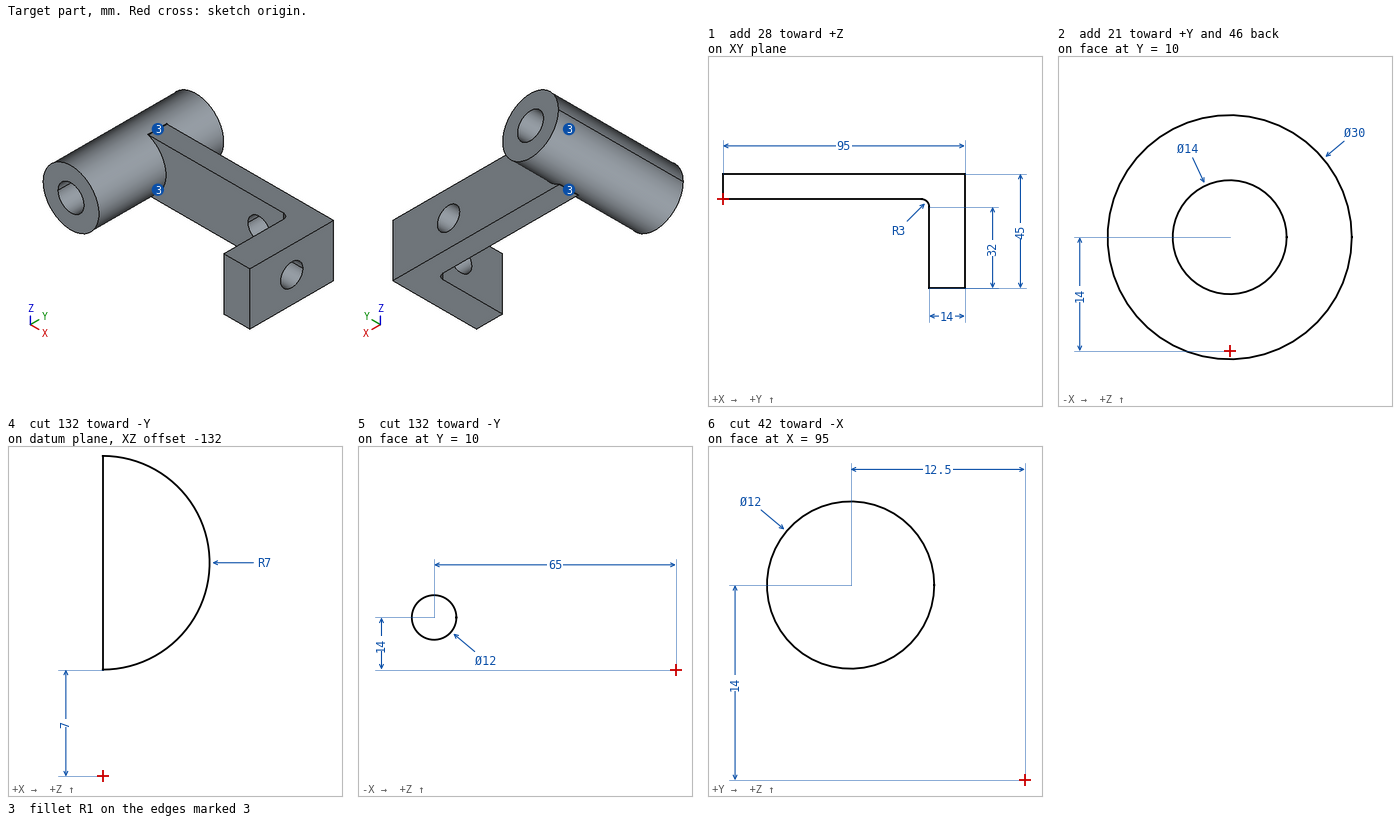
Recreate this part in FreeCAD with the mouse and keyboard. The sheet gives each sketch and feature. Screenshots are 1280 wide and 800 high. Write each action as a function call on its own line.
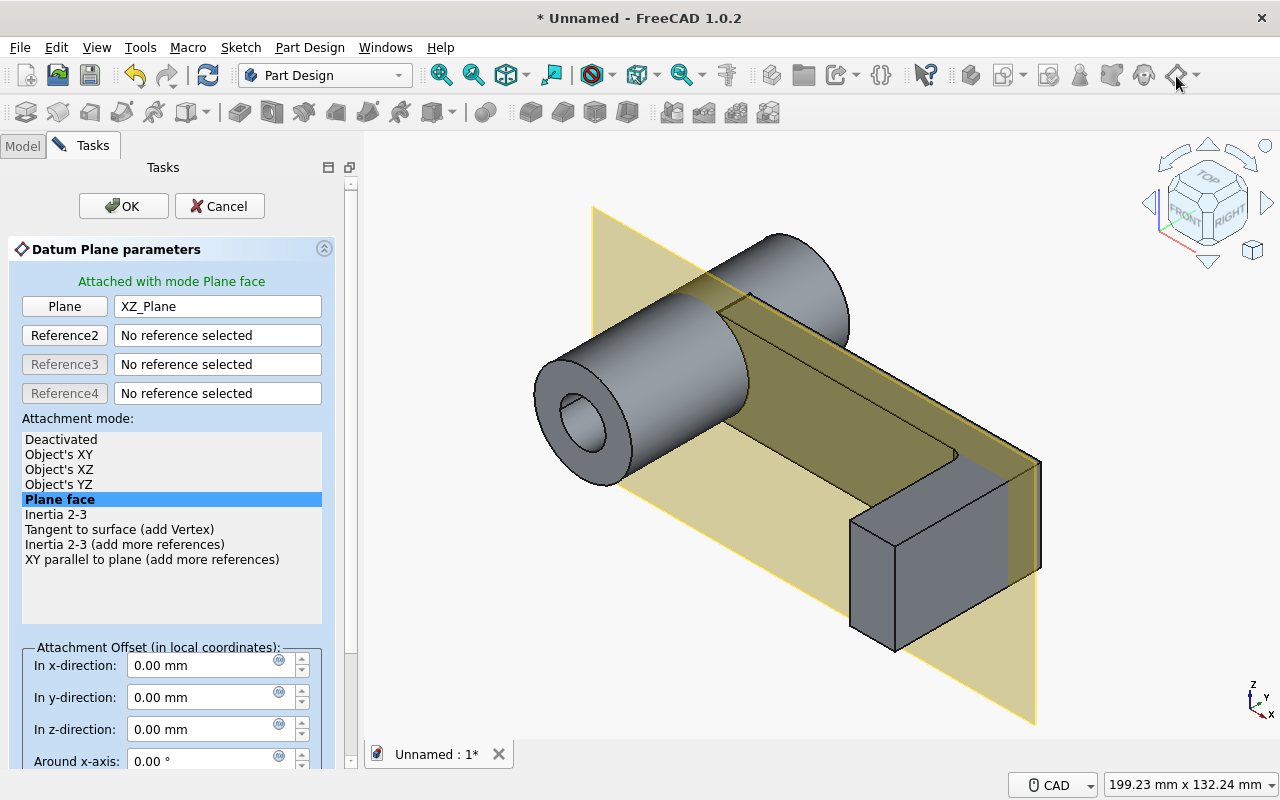
triple_click(210, 729)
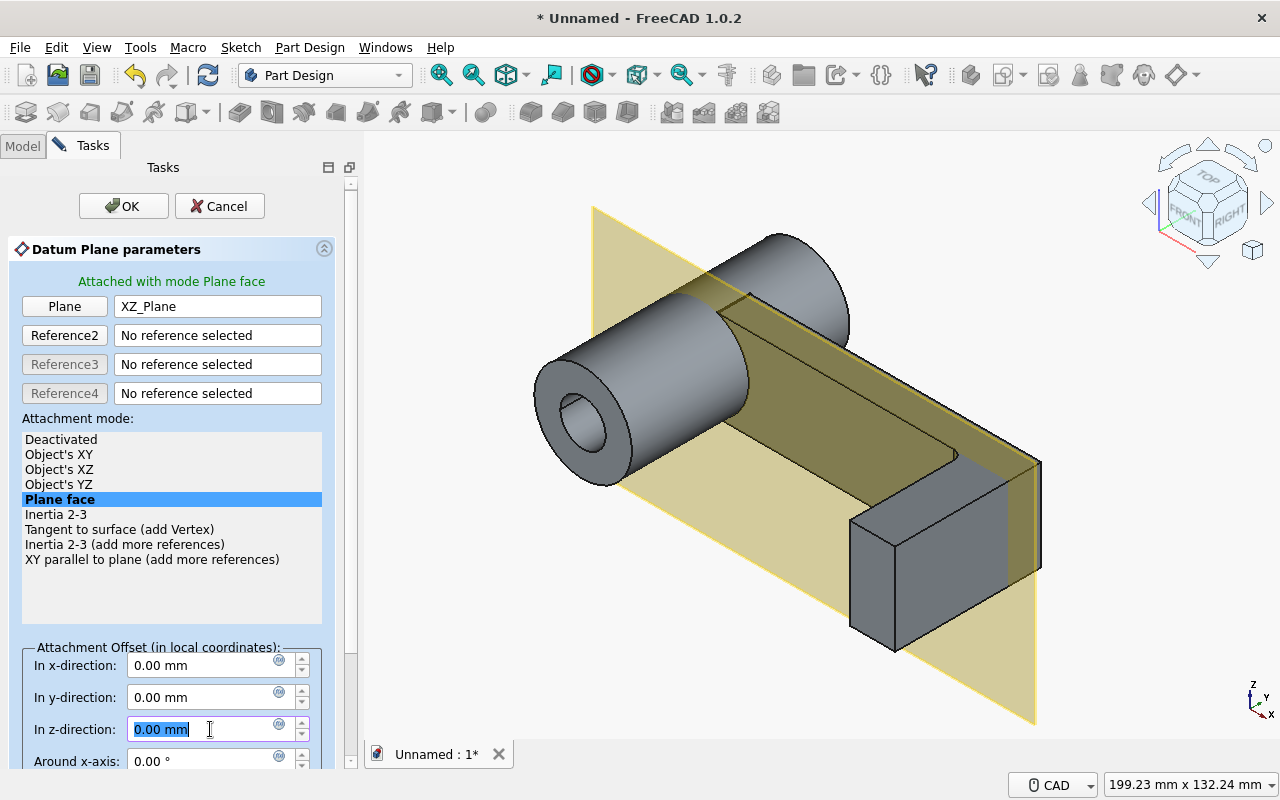
text(-132)
key(Tab)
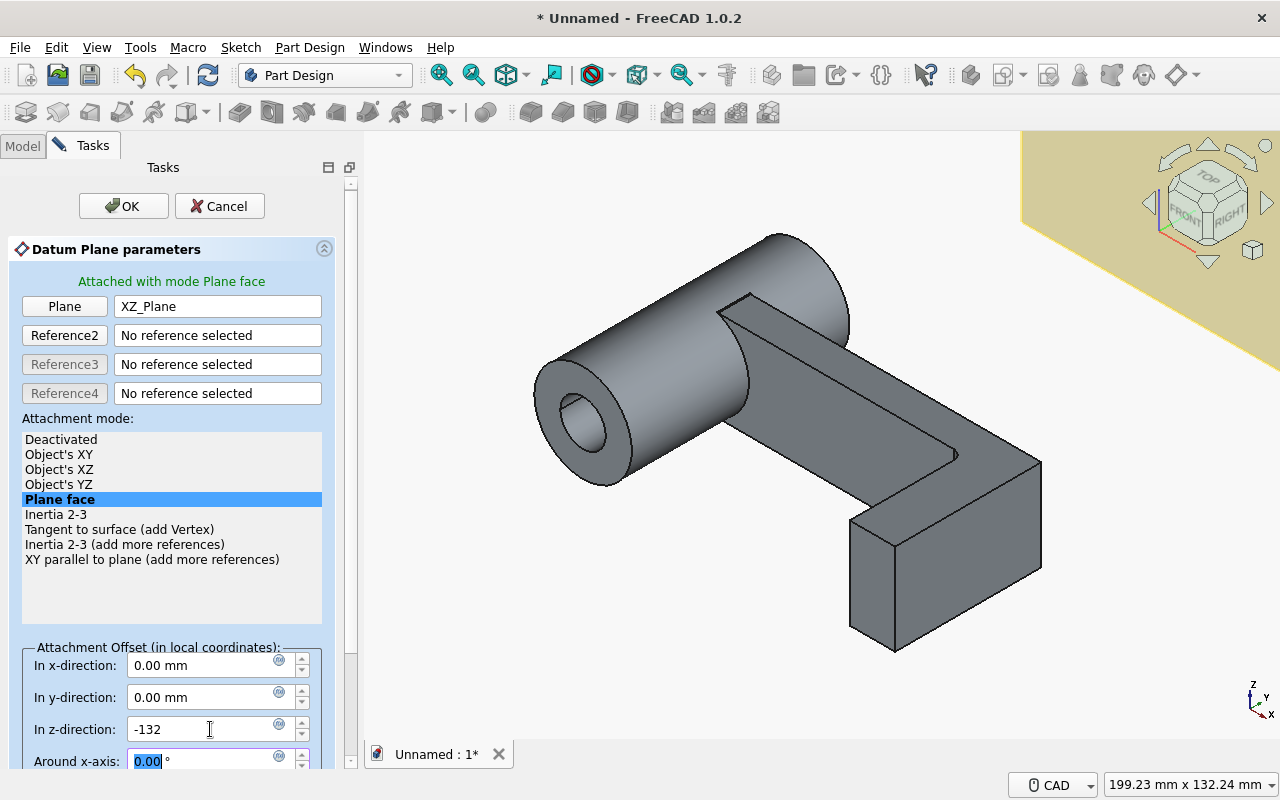
click(124, 206)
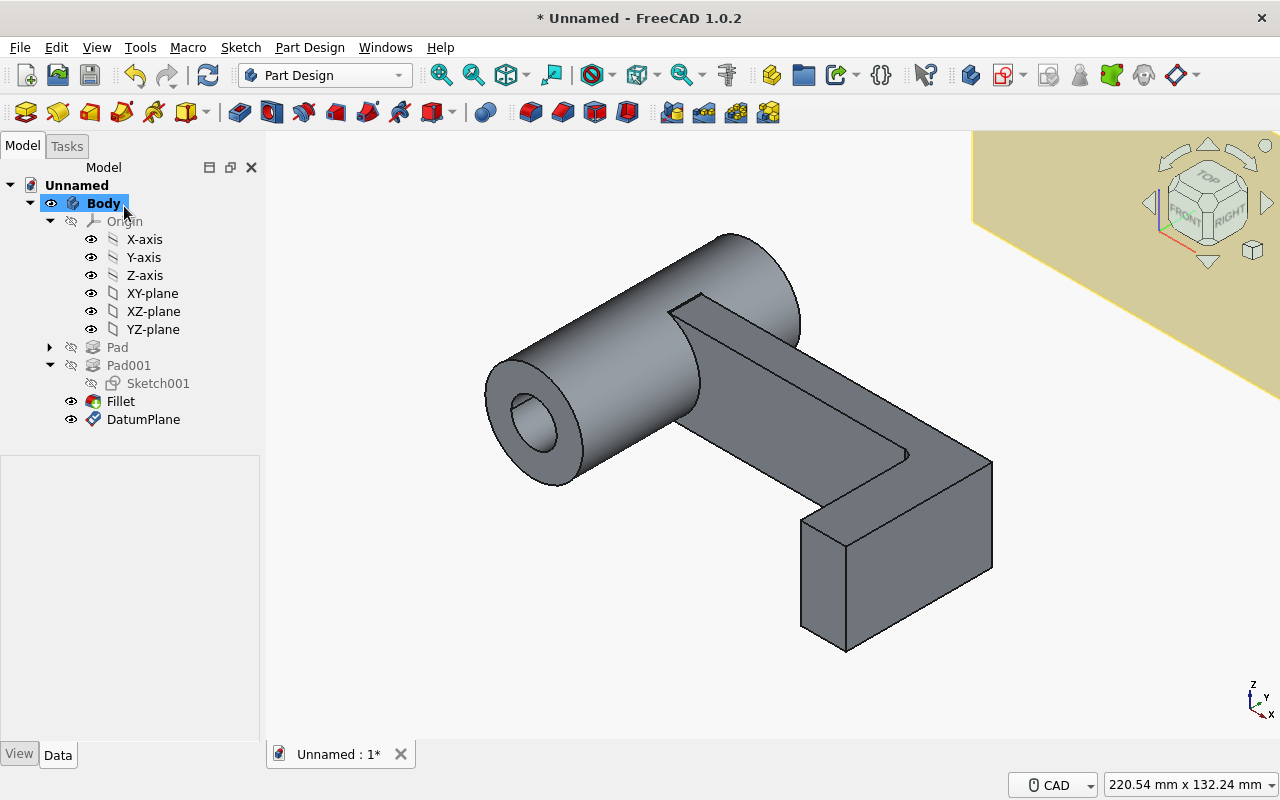
click(116, 419)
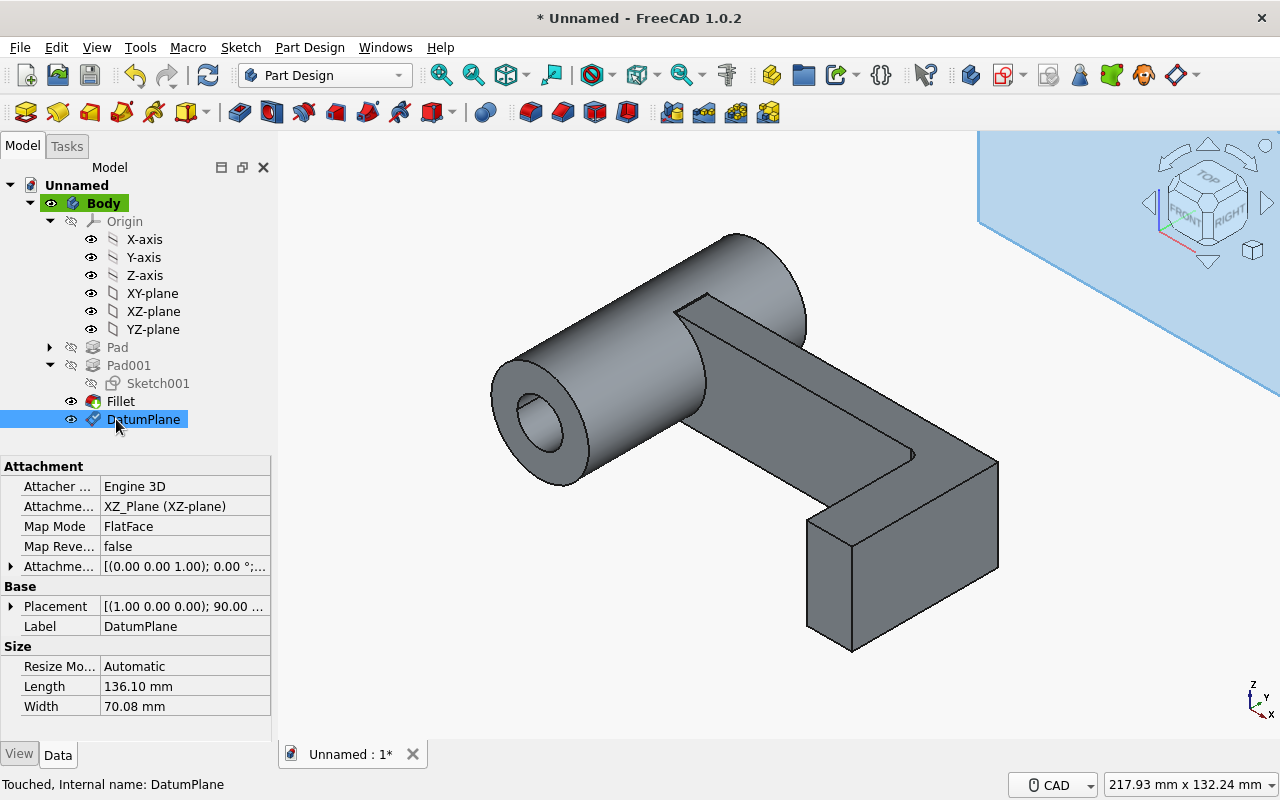
click(1004, 76)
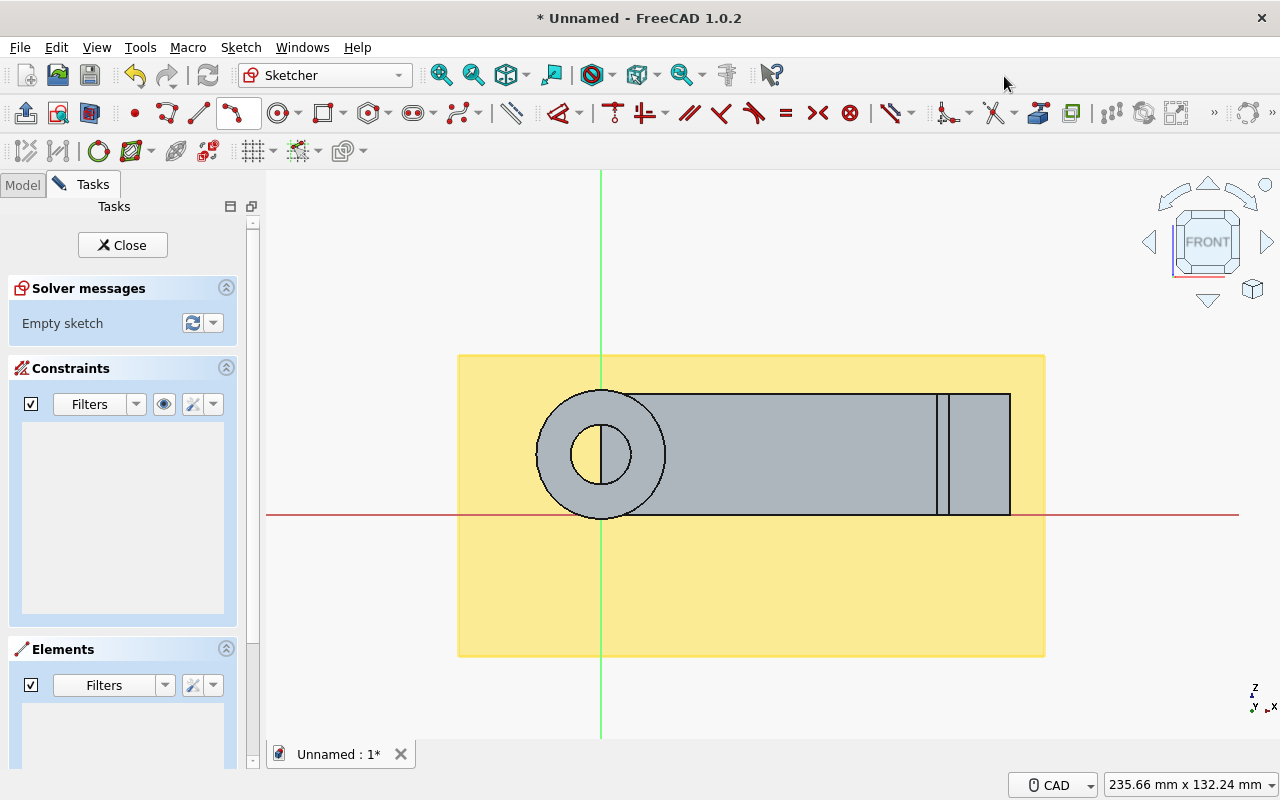
click(90, 114)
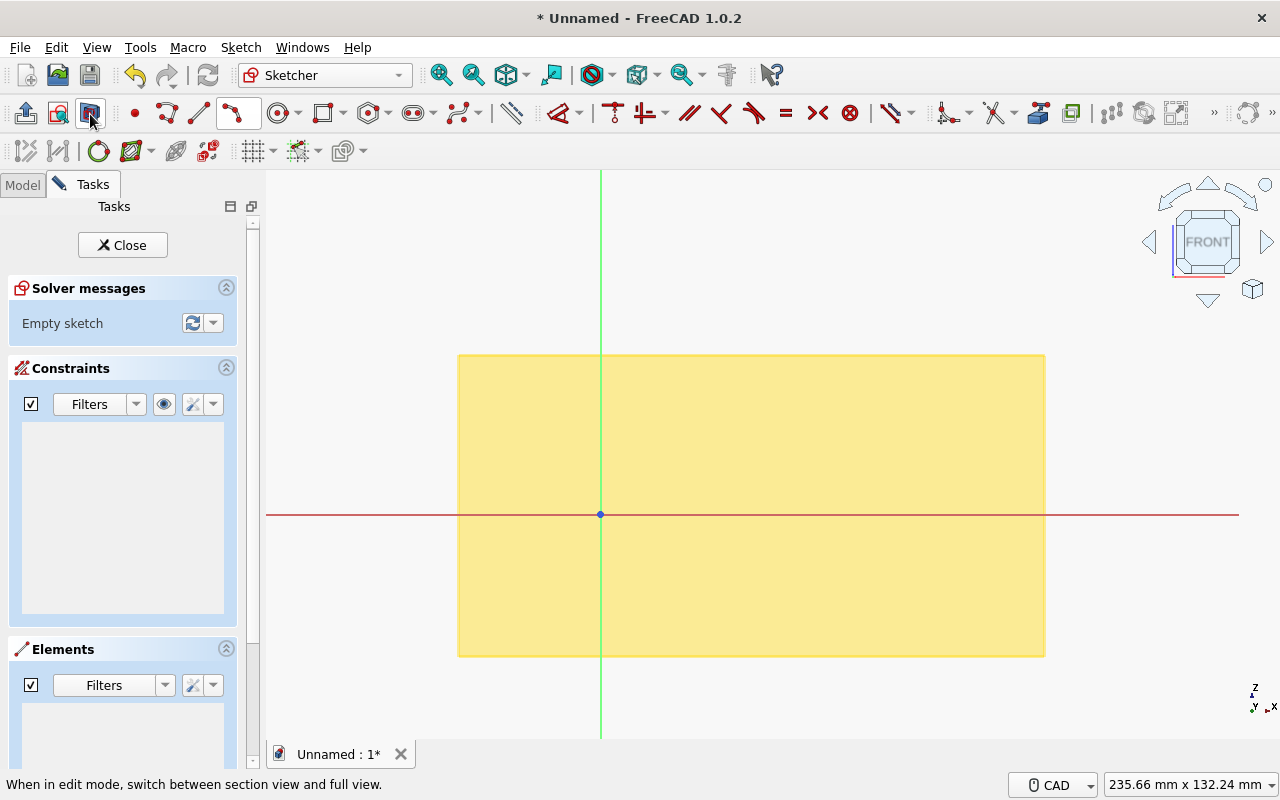
scroll(587, 474, up, 7)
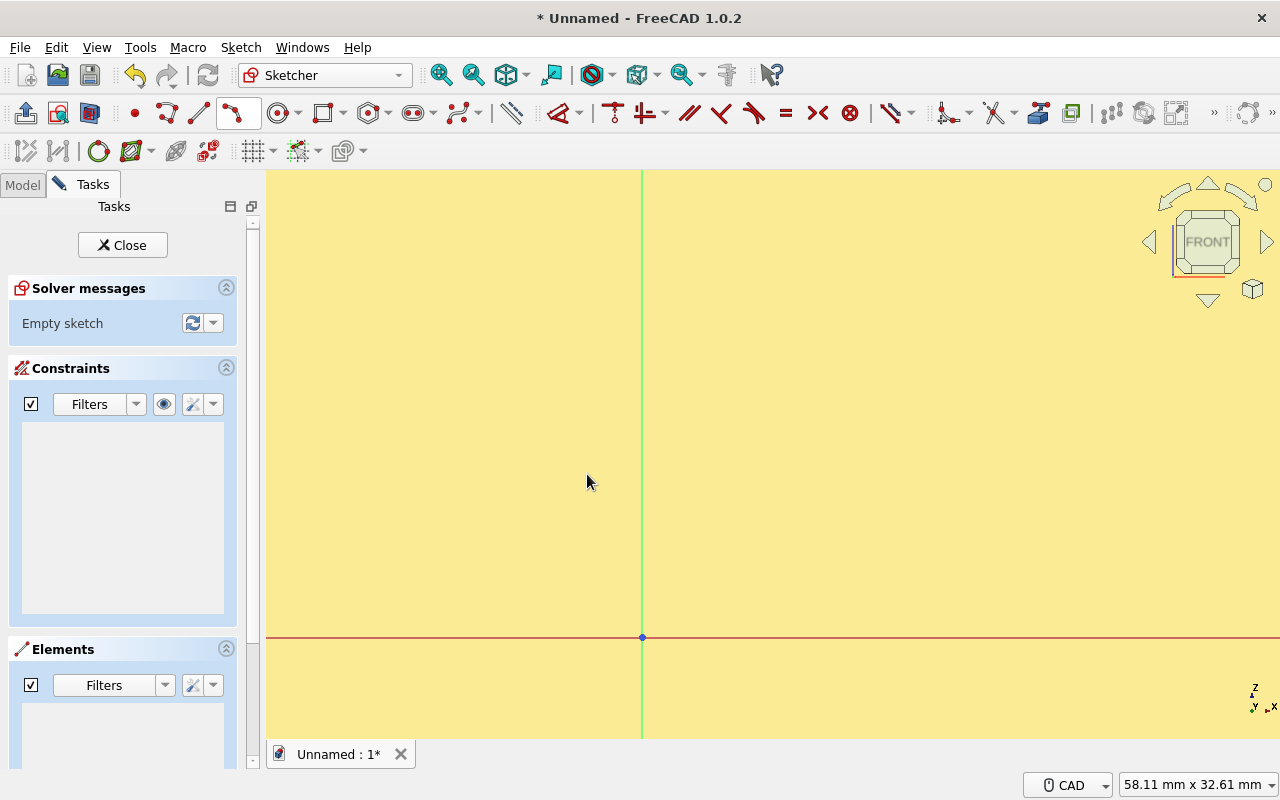
click(200, 114)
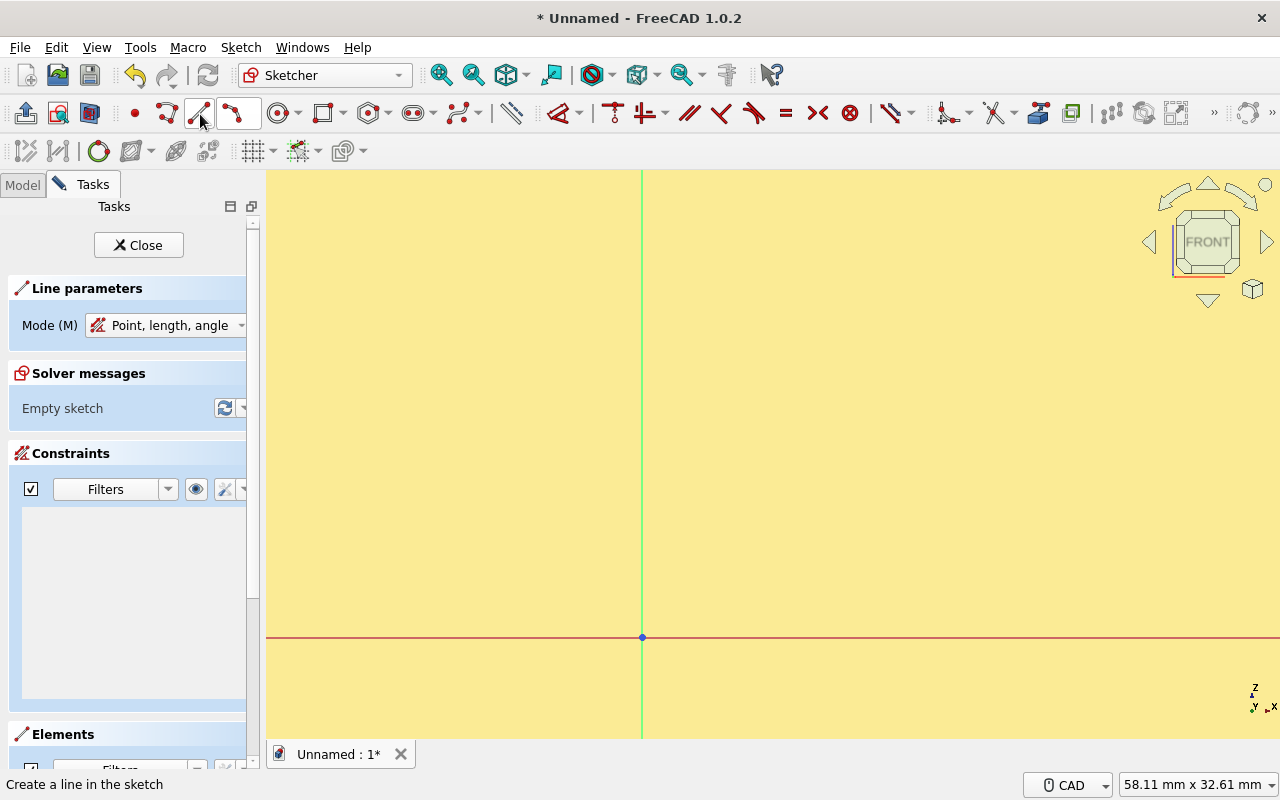
click(642, 515)
click(651, 271)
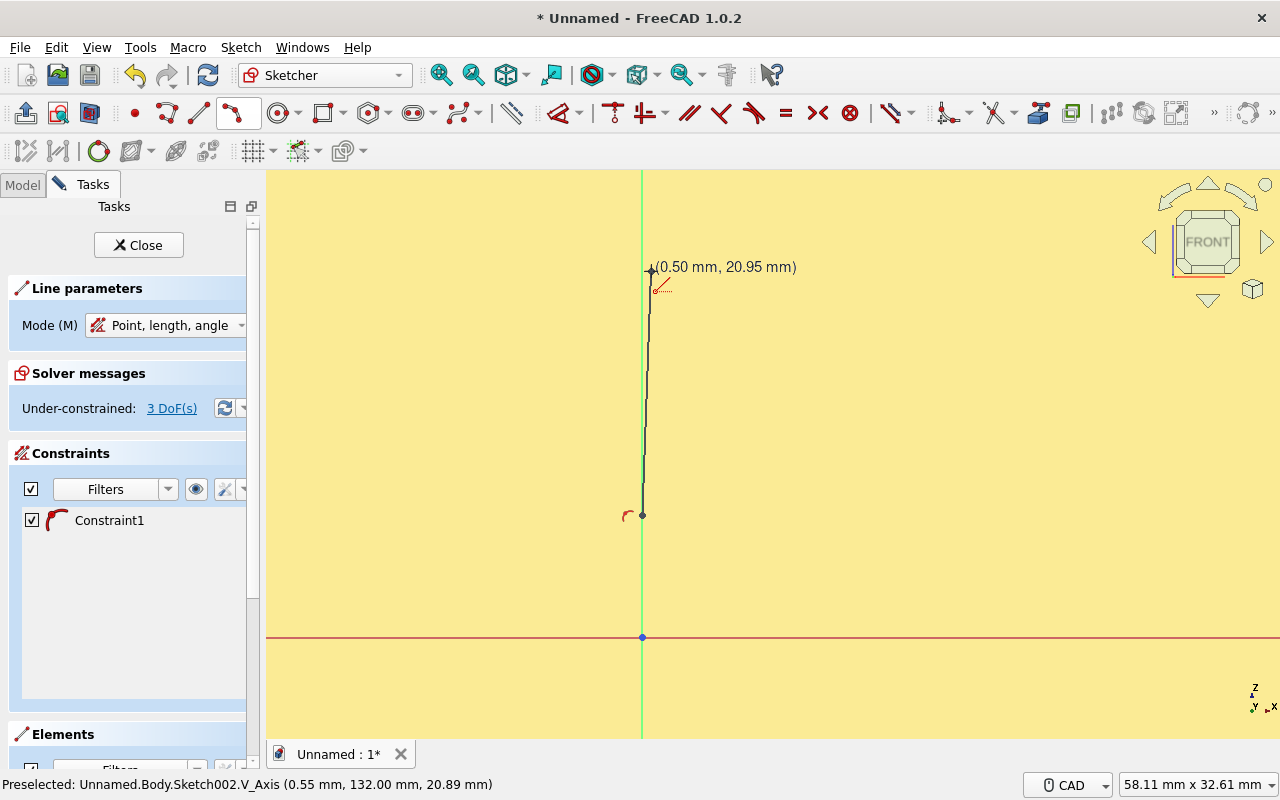
click(232, 114)